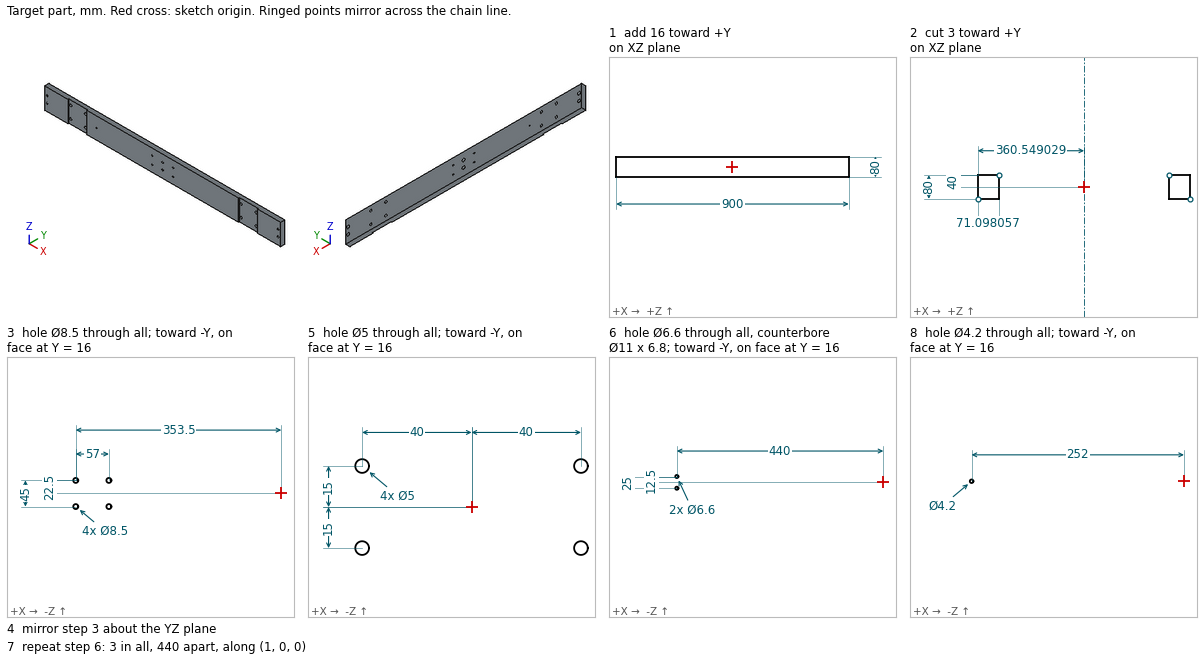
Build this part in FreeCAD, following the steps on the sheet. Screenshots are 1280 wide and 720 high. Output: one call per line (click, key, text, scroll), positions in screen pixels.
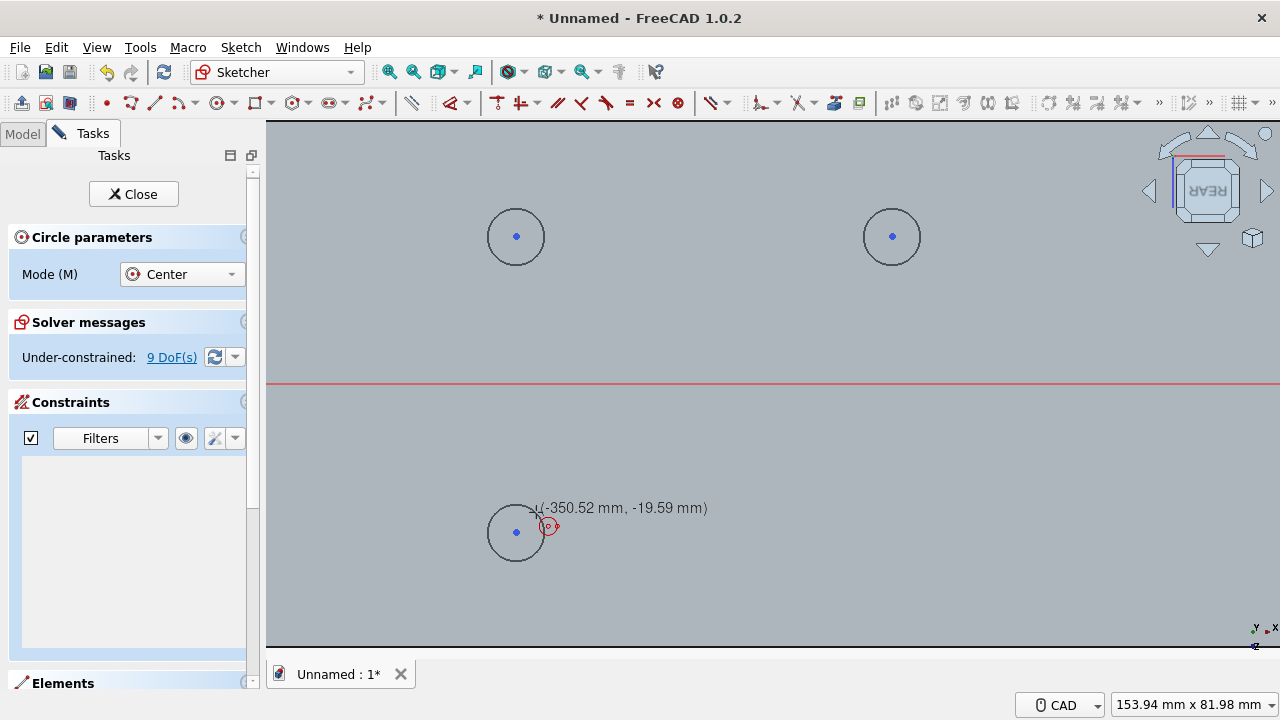
click(892, 532)
click(912, 512)
key(Escape)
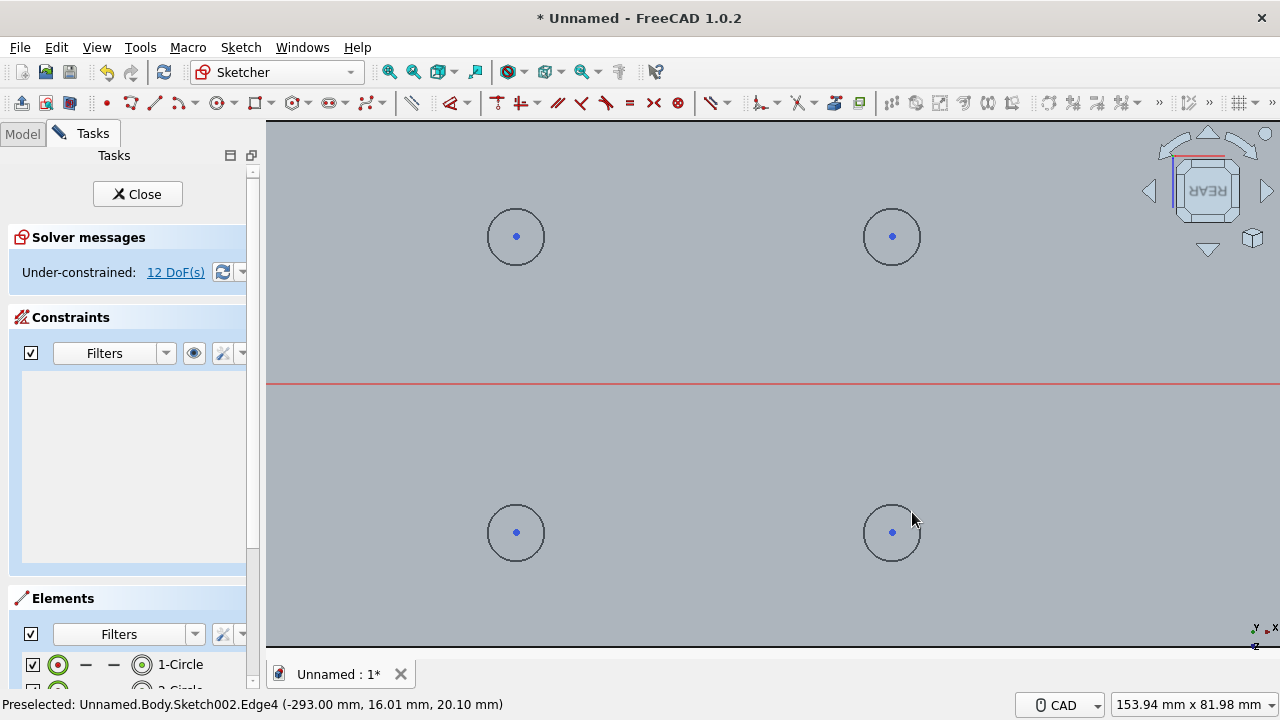
click(536, 217)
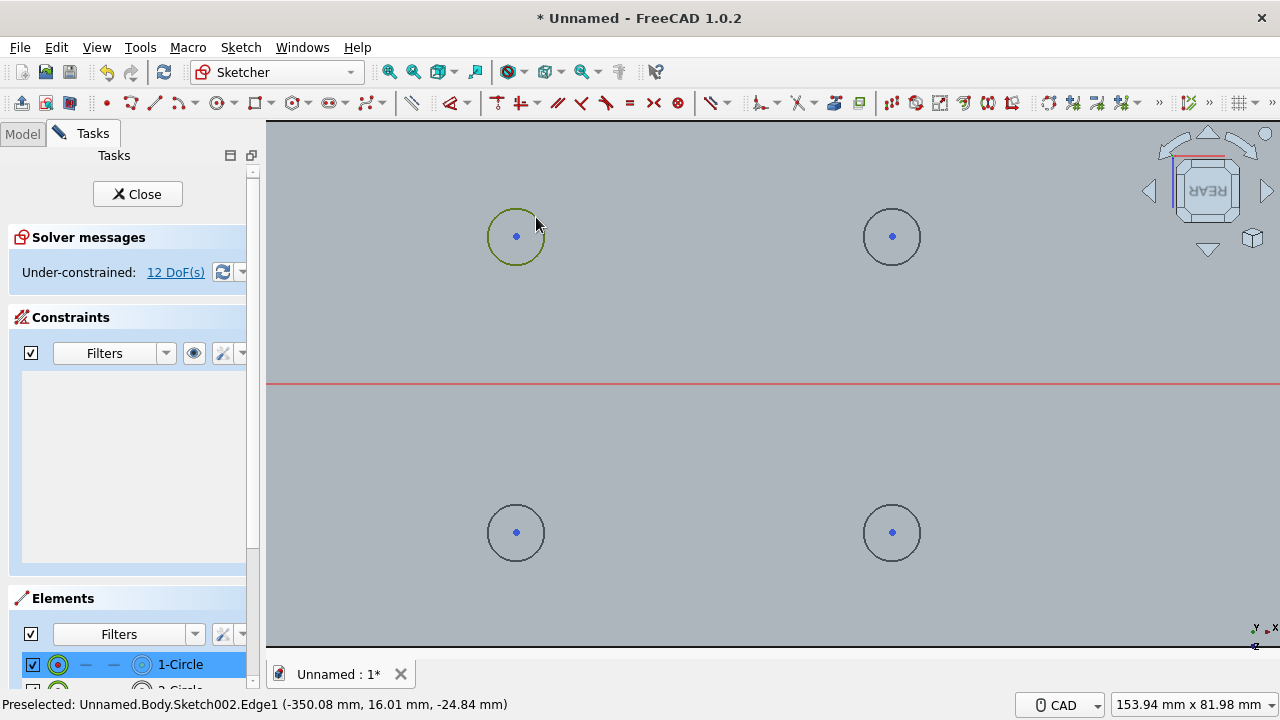
click(912, 217)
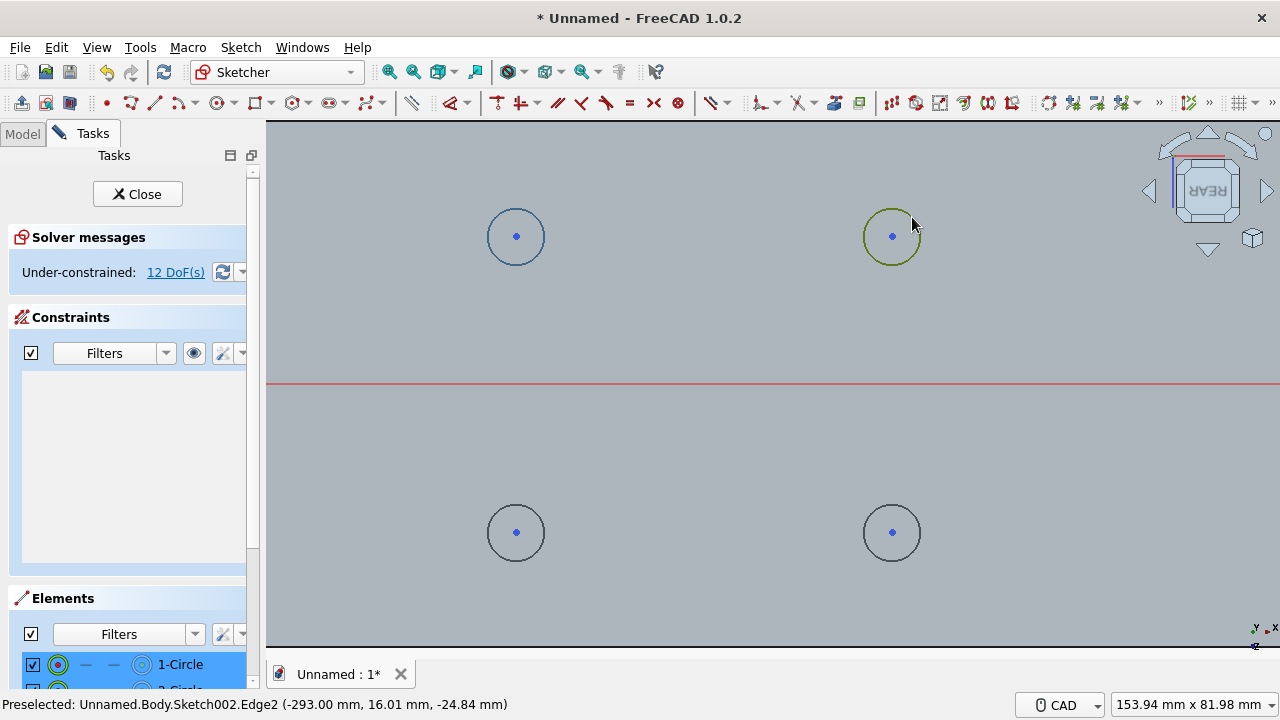
click(536, 513)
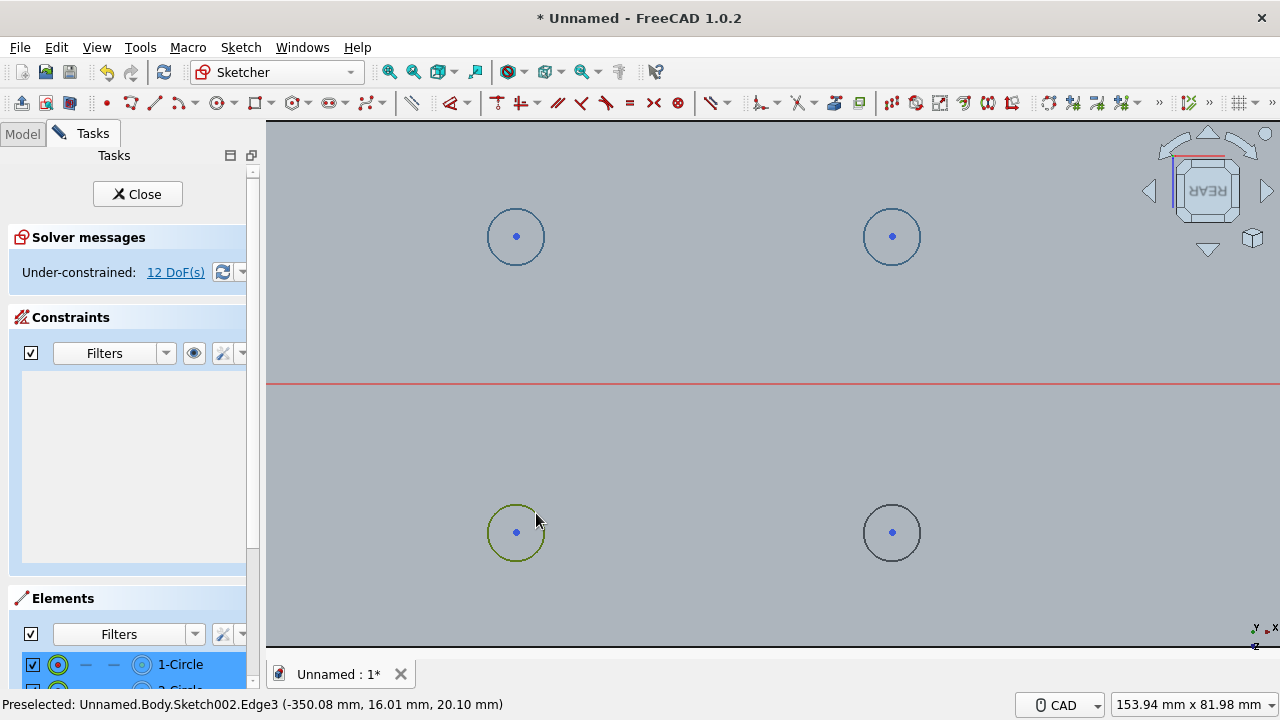
click(912, 513)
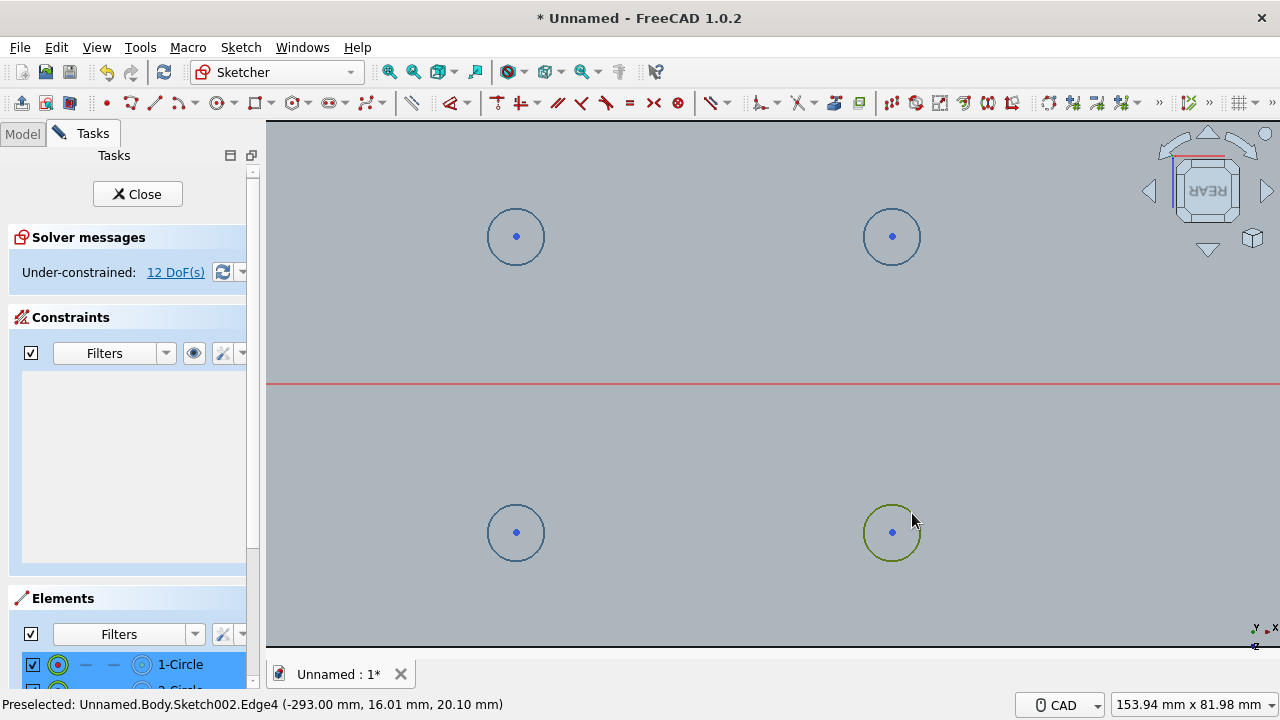
key(e)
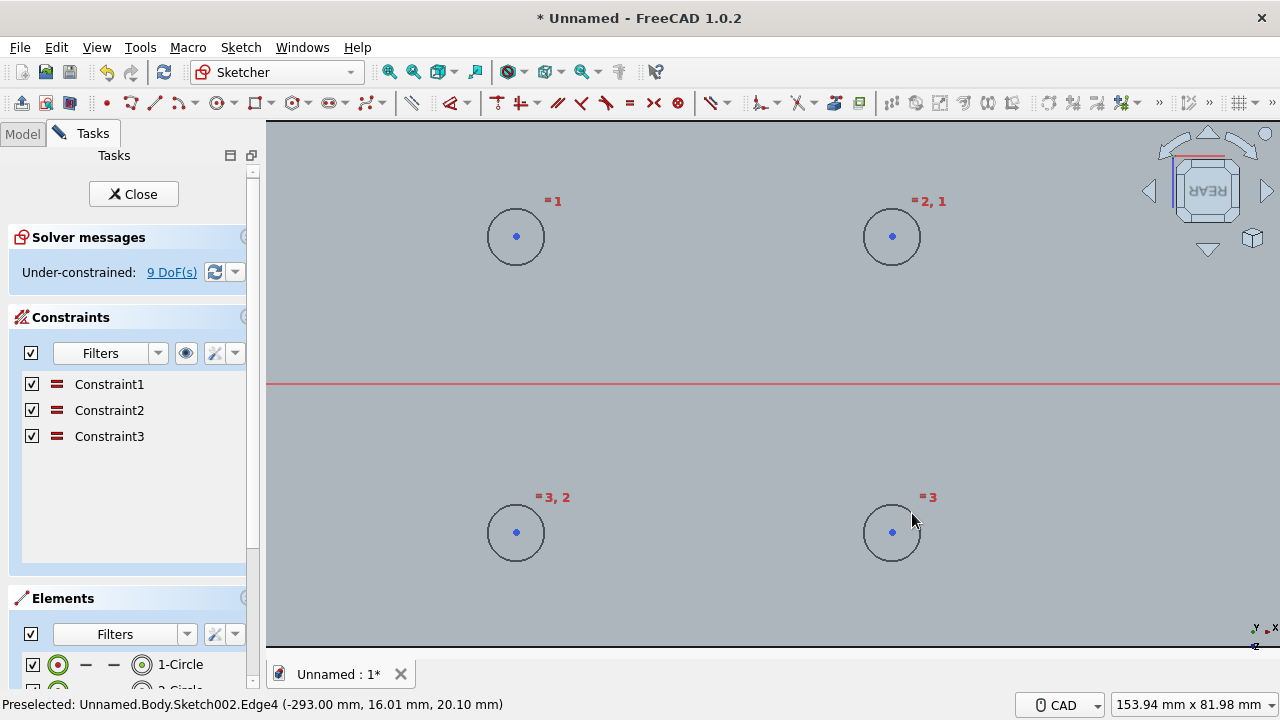
click(516, 237)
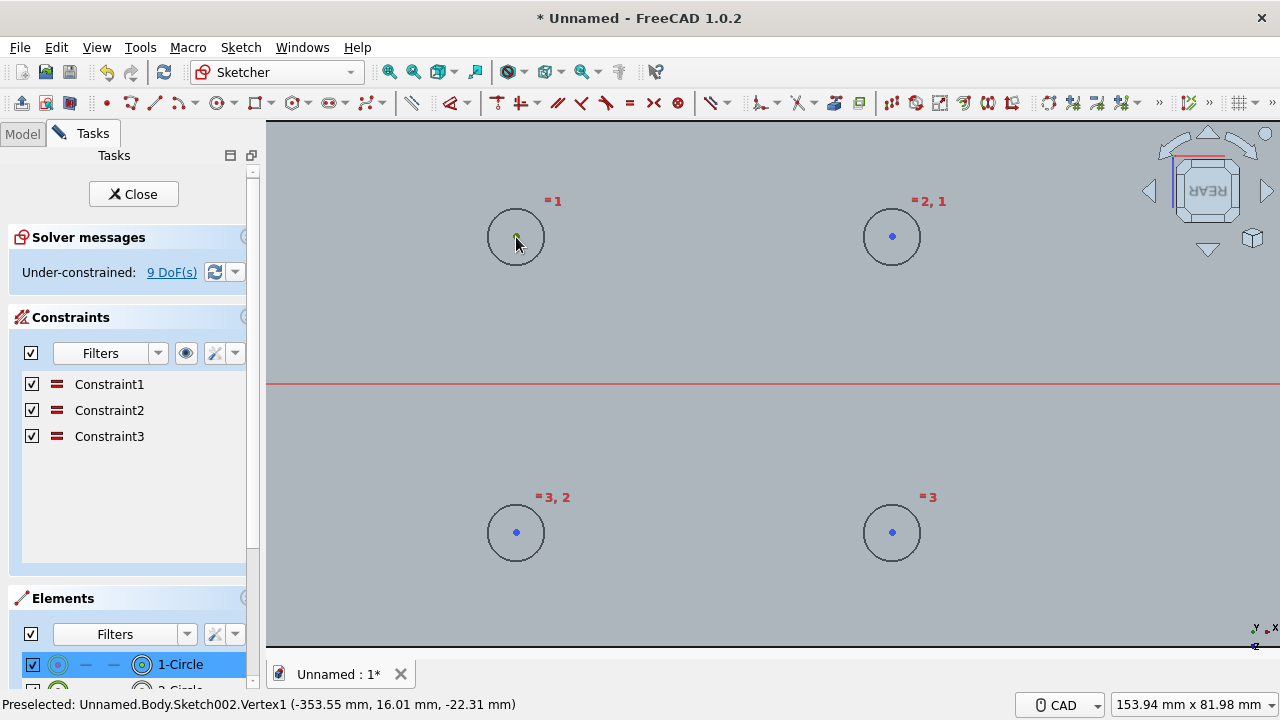
click(892, 237)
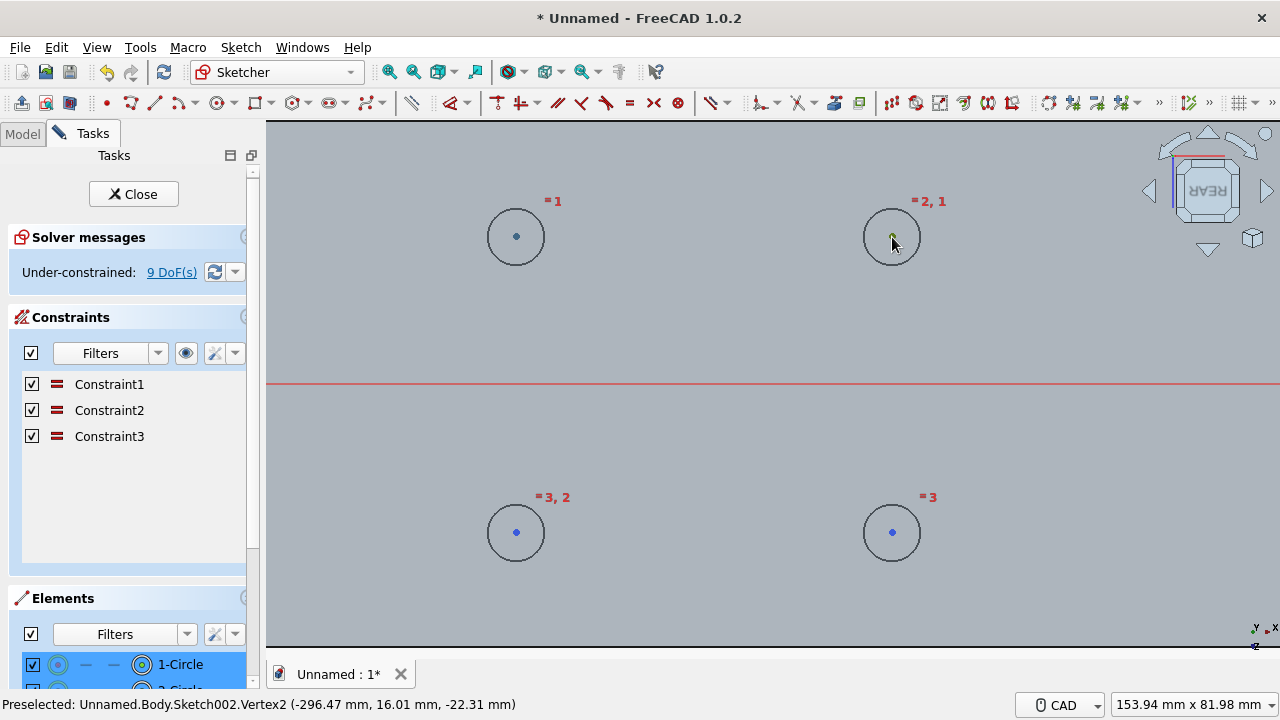
key(h)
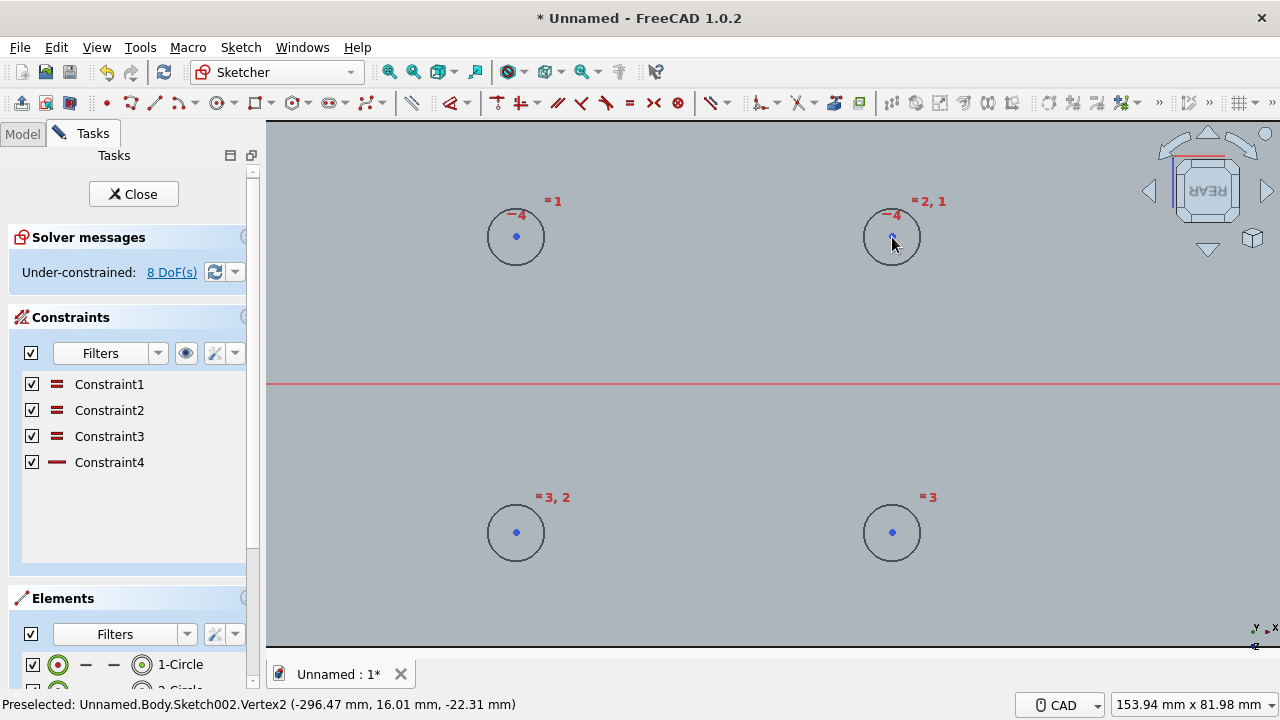
click(516, 237)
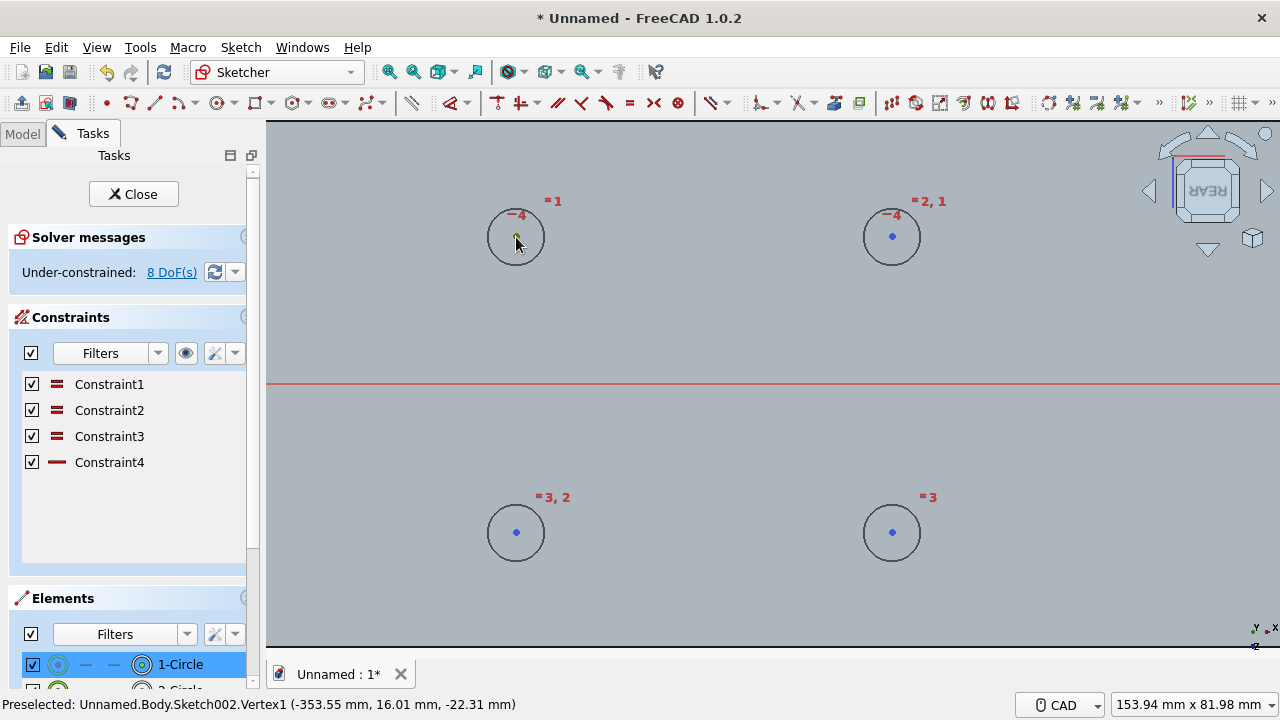
click(516, 533)